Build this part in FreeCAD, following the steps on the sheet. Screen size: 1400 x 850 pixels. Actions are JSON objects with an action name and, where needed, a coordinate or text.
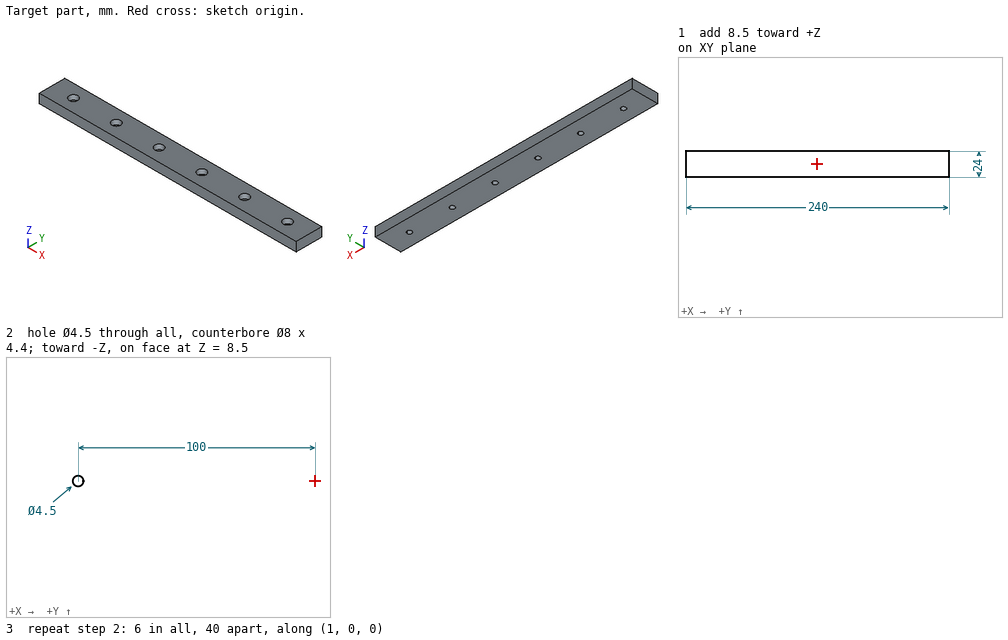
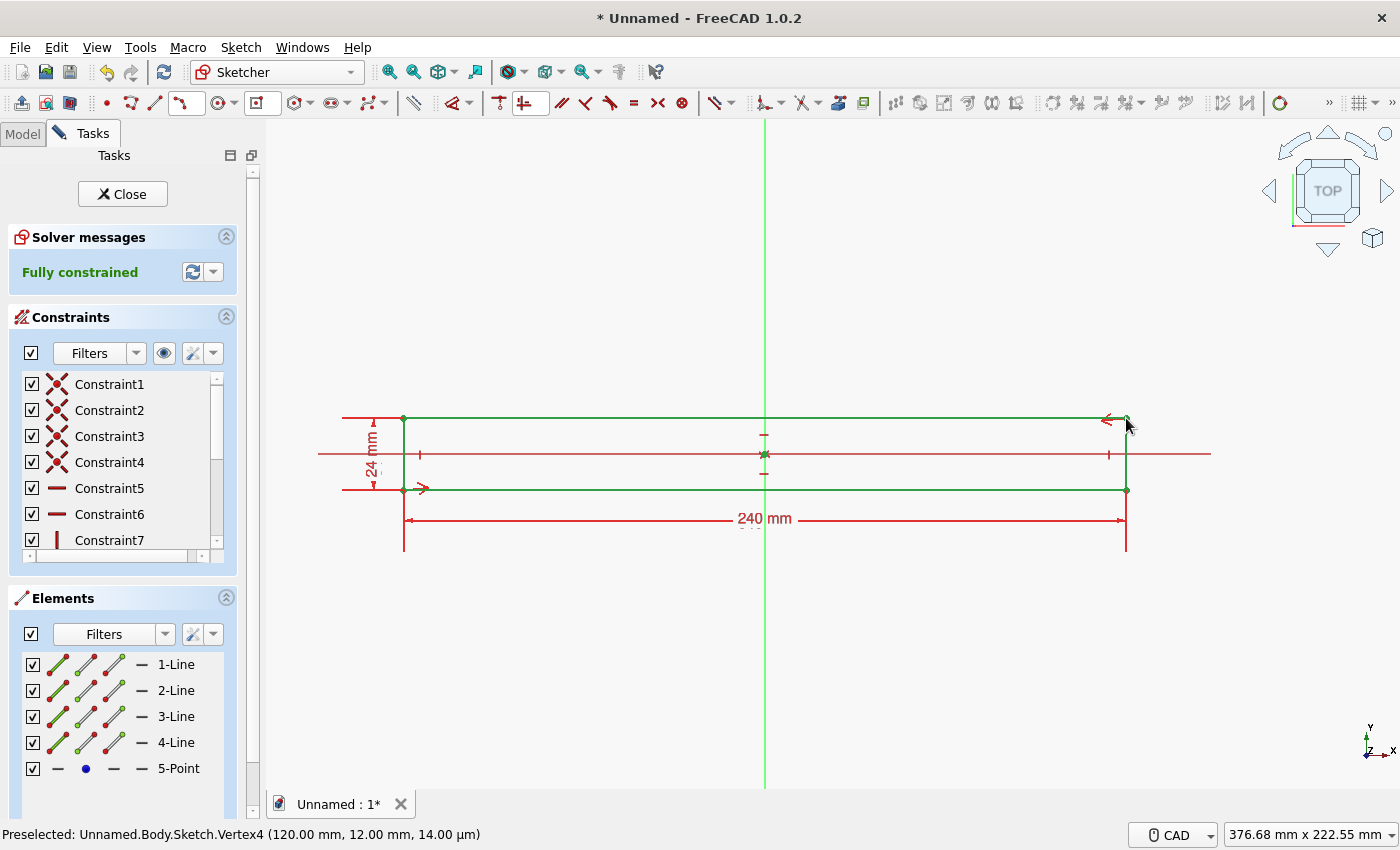
{"action": "left_click", "coordinate": [123, 194]}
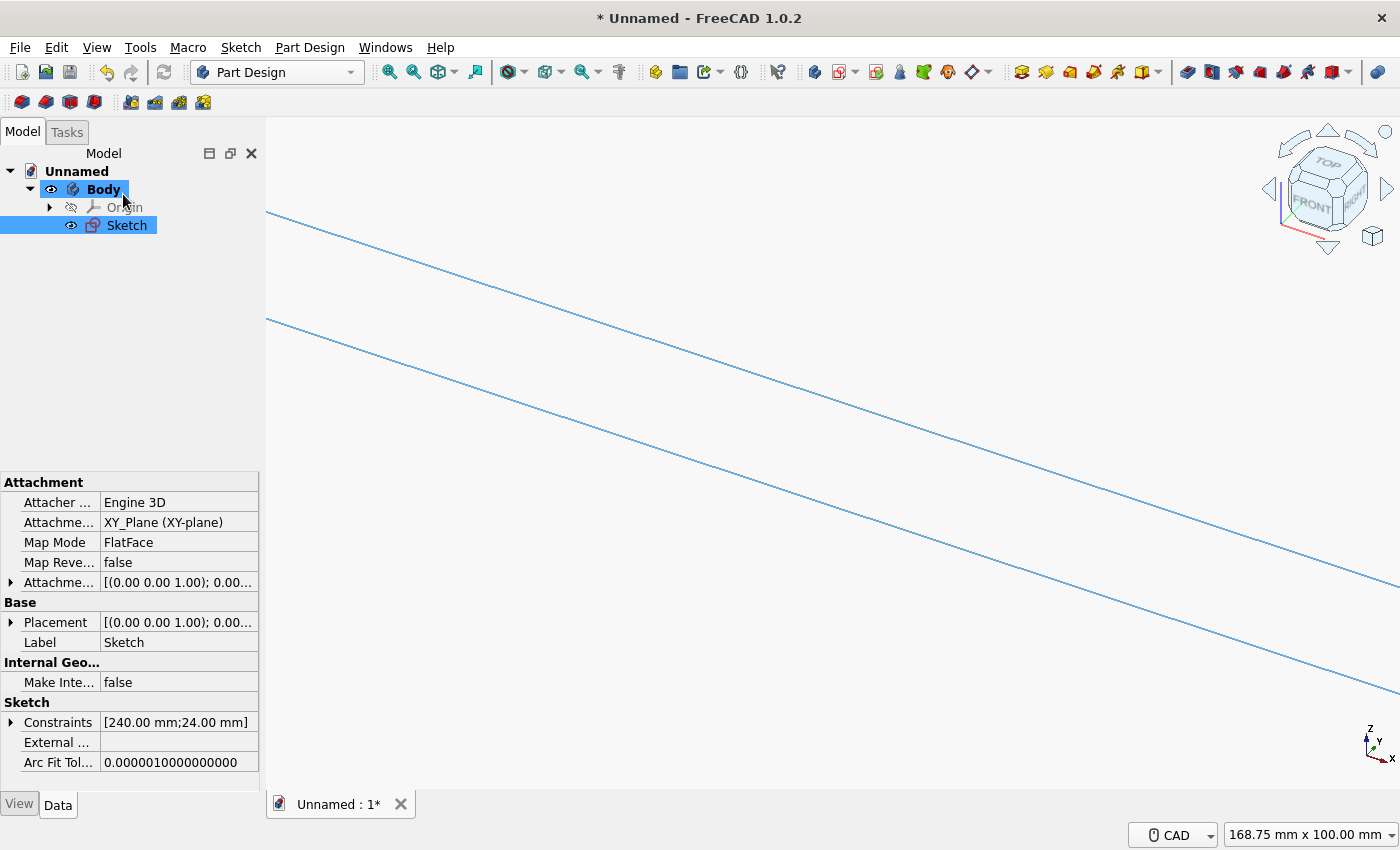
{"action": "left_click", "coordinate": [1022, 72]}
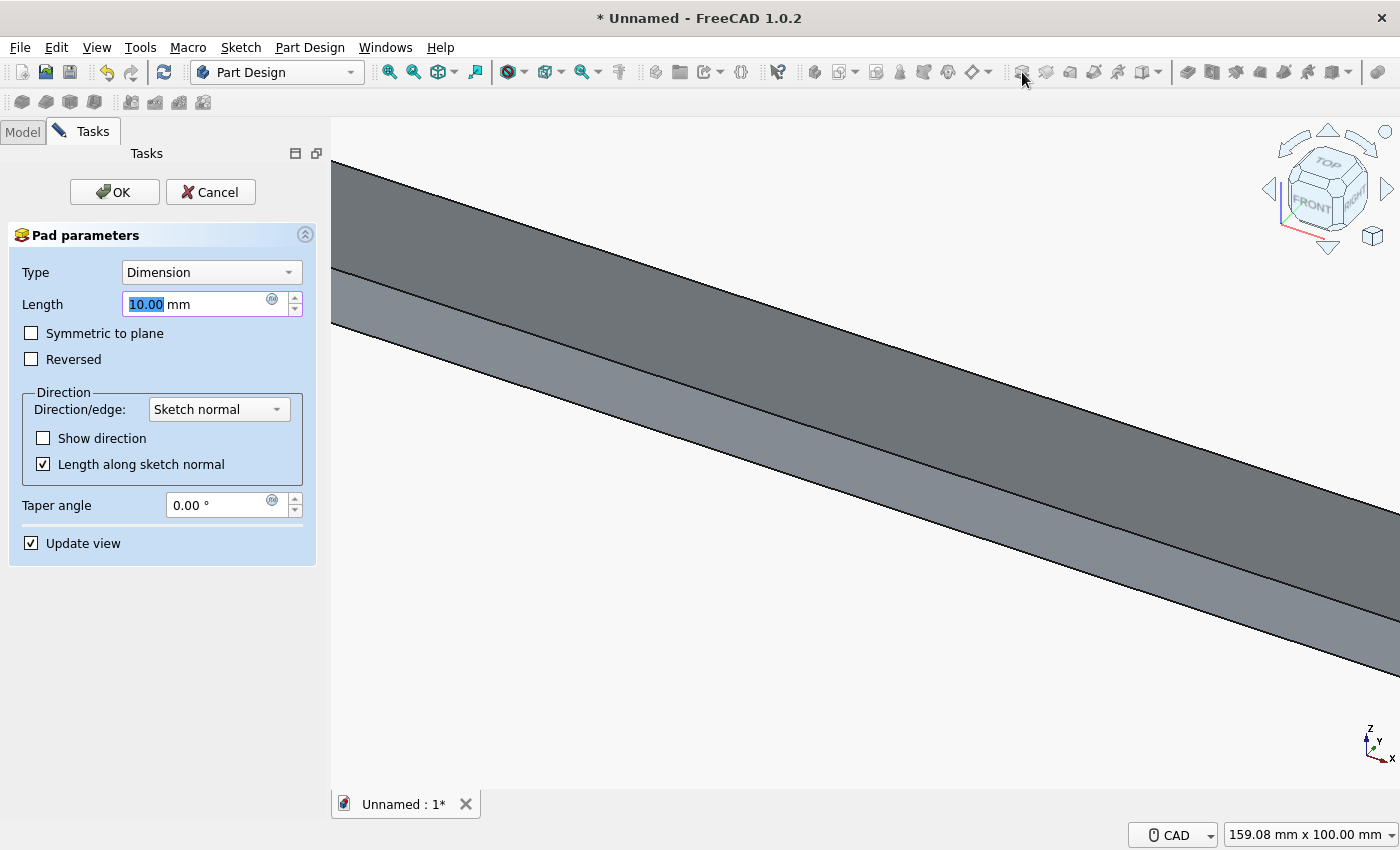
{"action": "type", "text": "8.5"}
{"action": "key", "text": "Tab"}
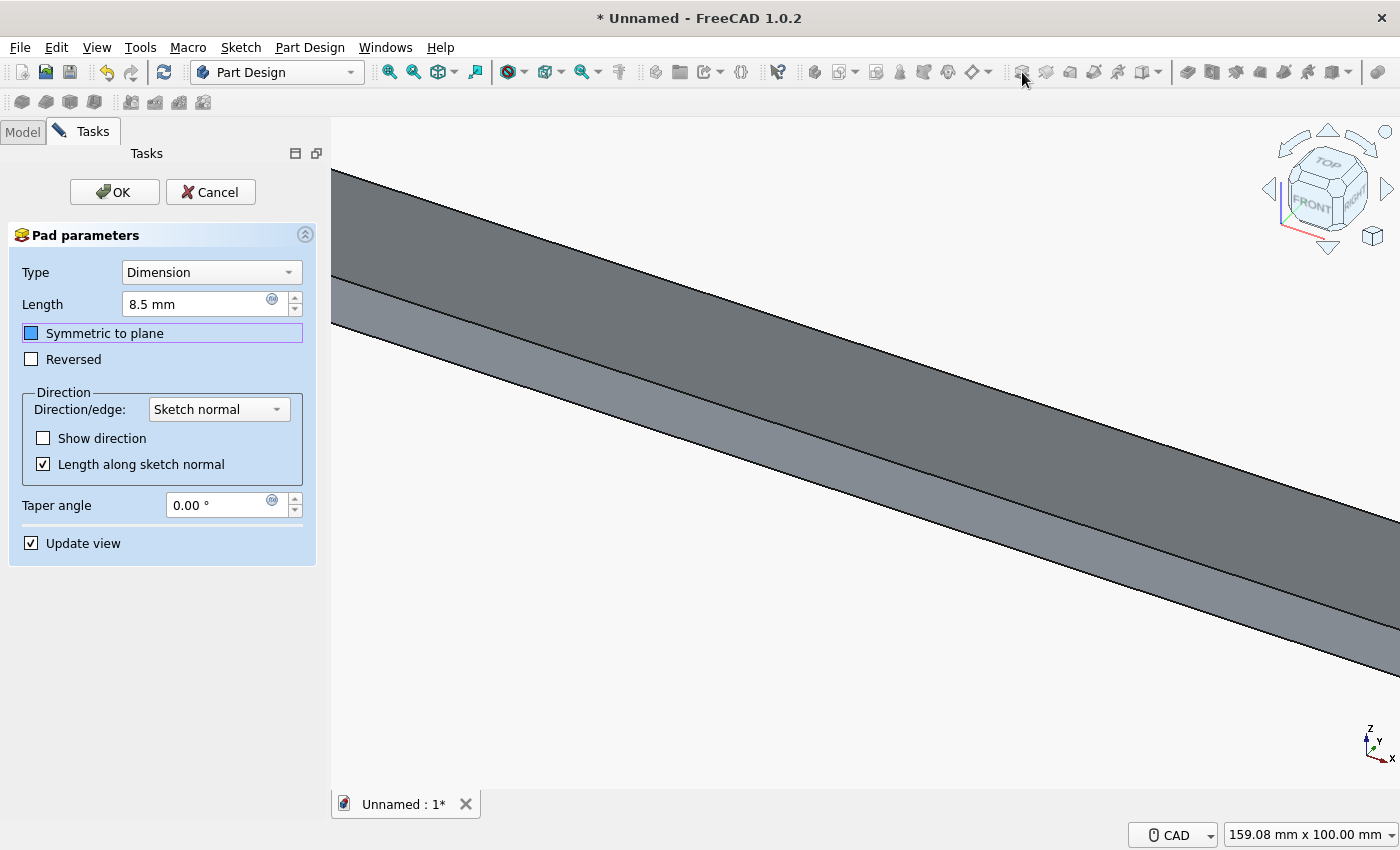
{"action": "left_click", "coordinate": [115, 192]}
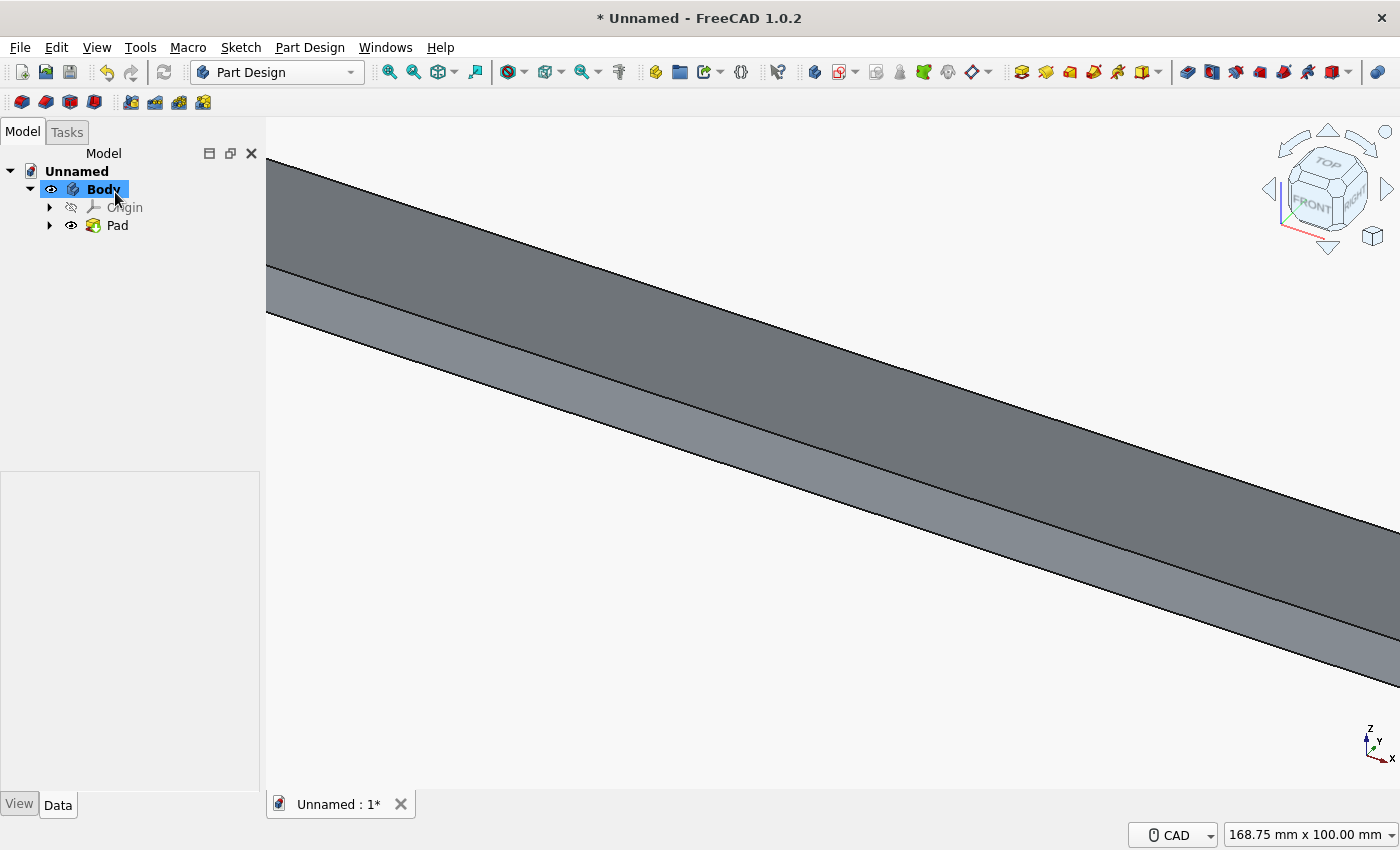
{"action": "key", "text": "v f"}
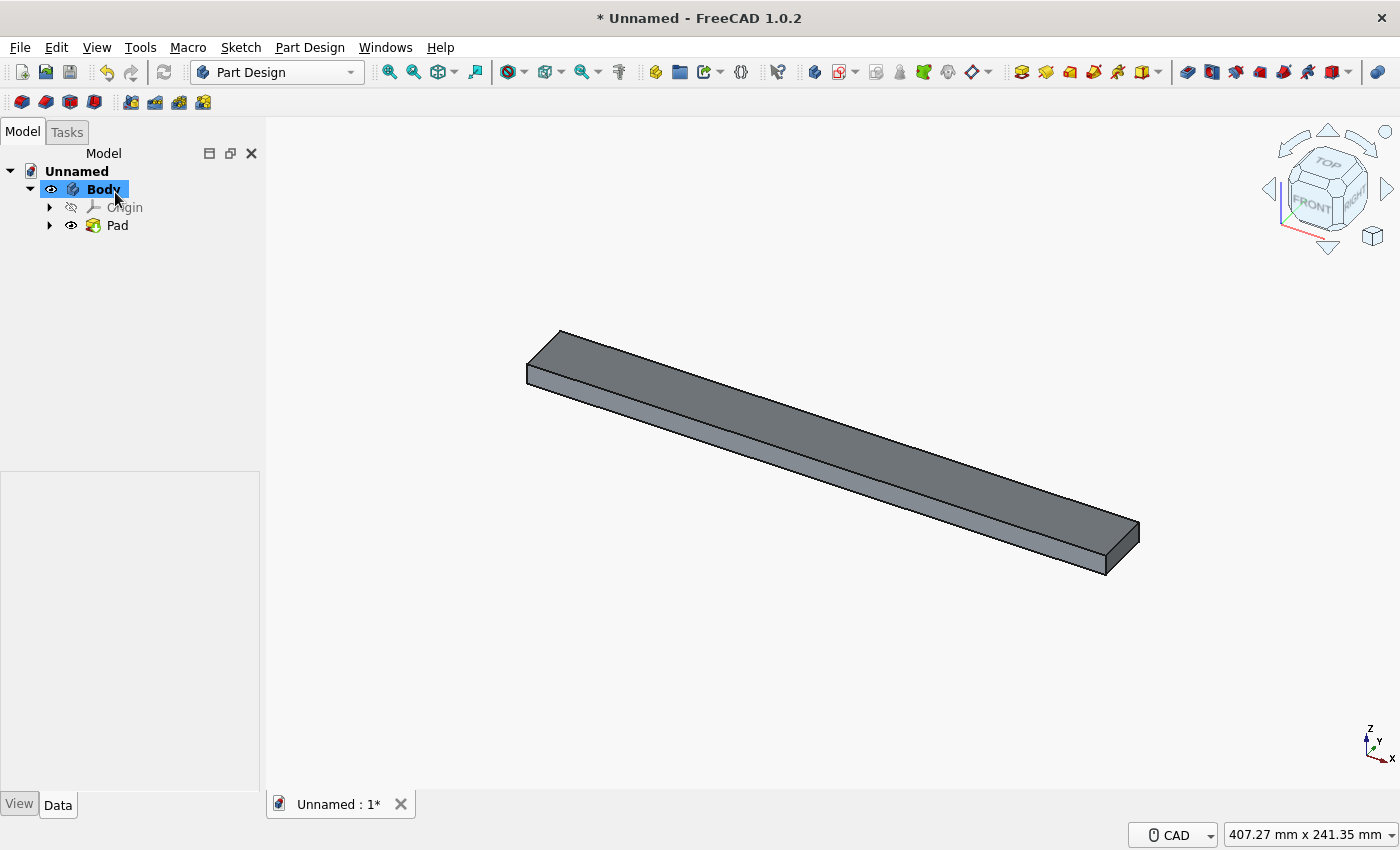
{"action": "left_click", "coordinate": [1081, 524]}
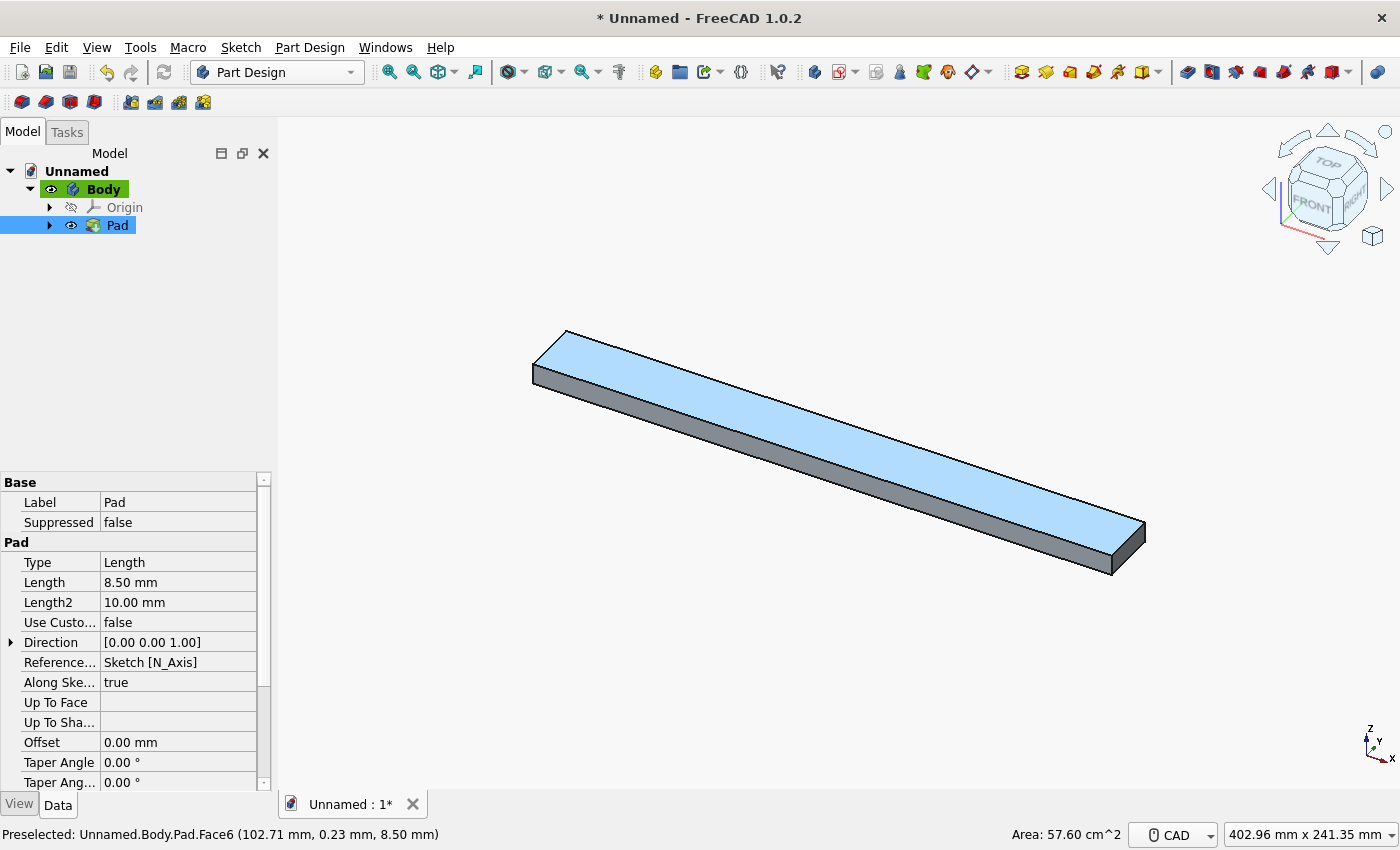
{"action": "left_click", "coordinate": [840, 72]}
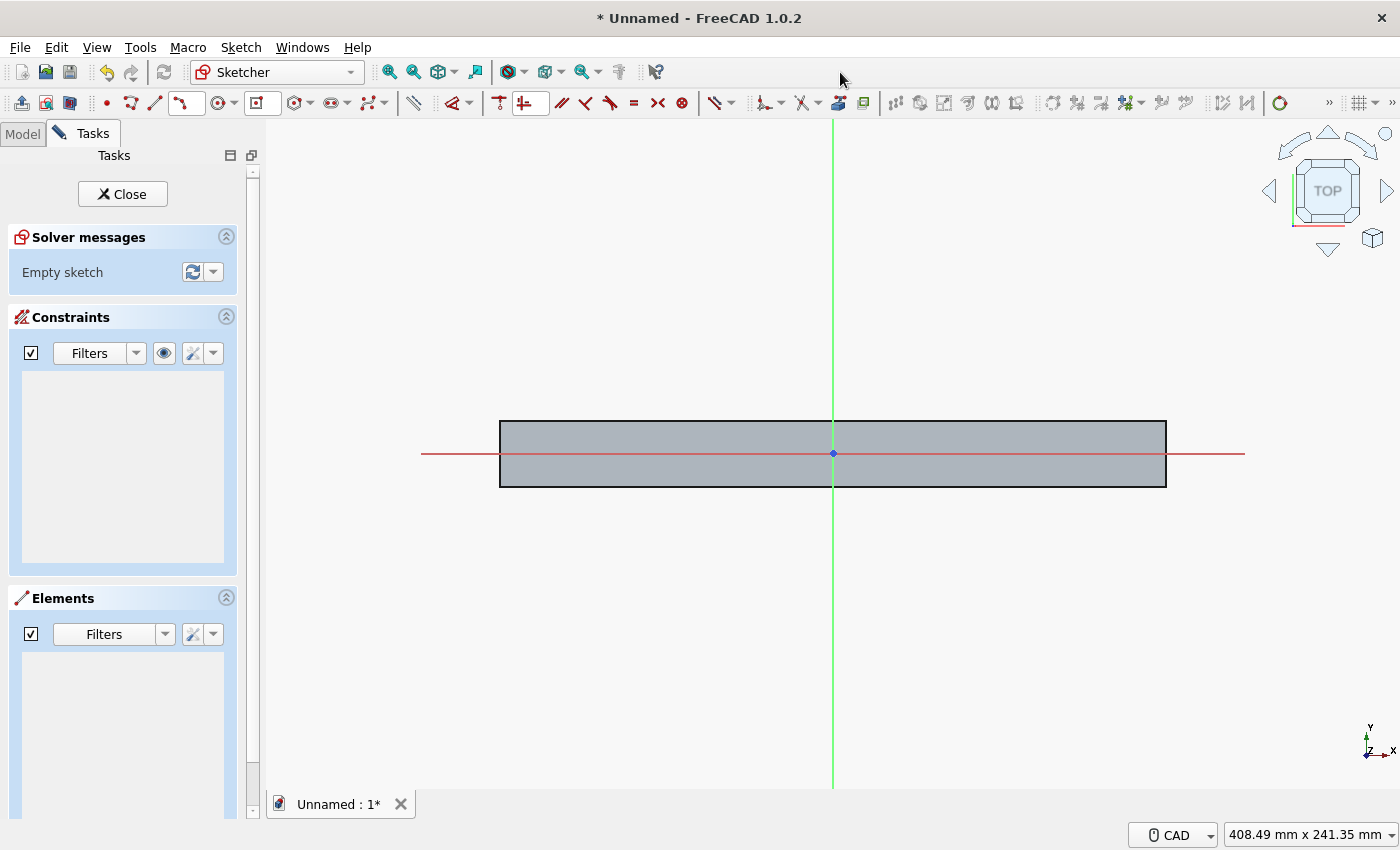
{"action": "scroll", "coordinate": [544, 454], "scroll_direction": "up", "scroll_amount": 15}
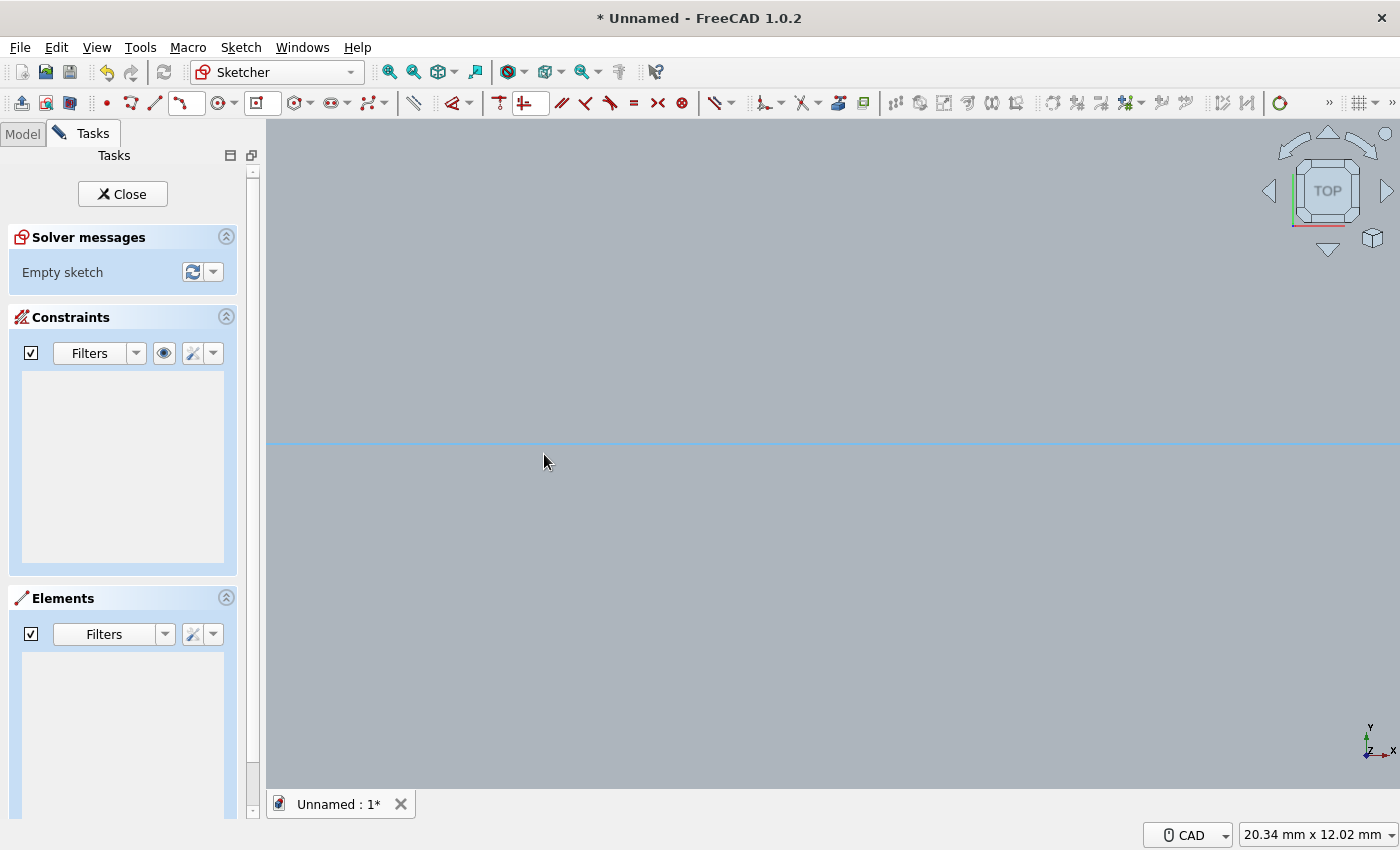
{"action": "scroll", "coordinate": [773, 433], "scroll_direction": "up", "scroll_amount": 3}